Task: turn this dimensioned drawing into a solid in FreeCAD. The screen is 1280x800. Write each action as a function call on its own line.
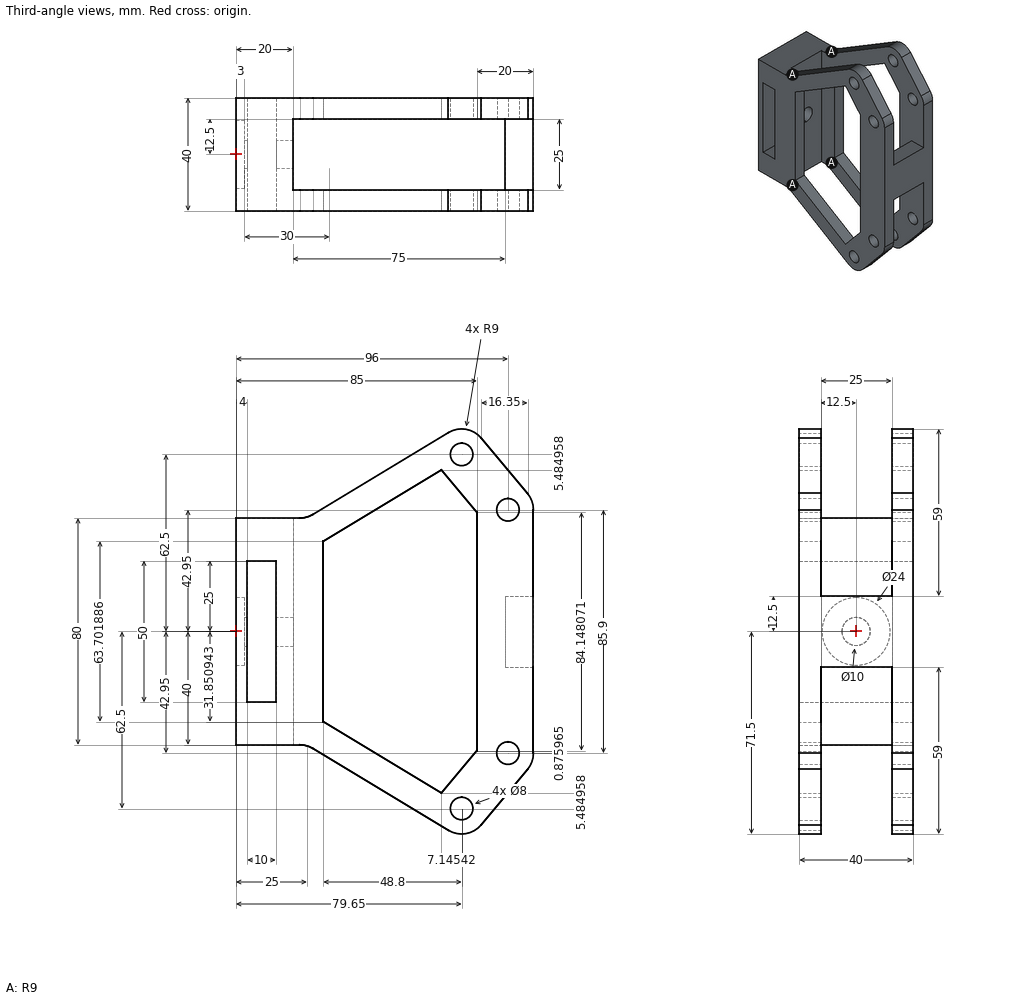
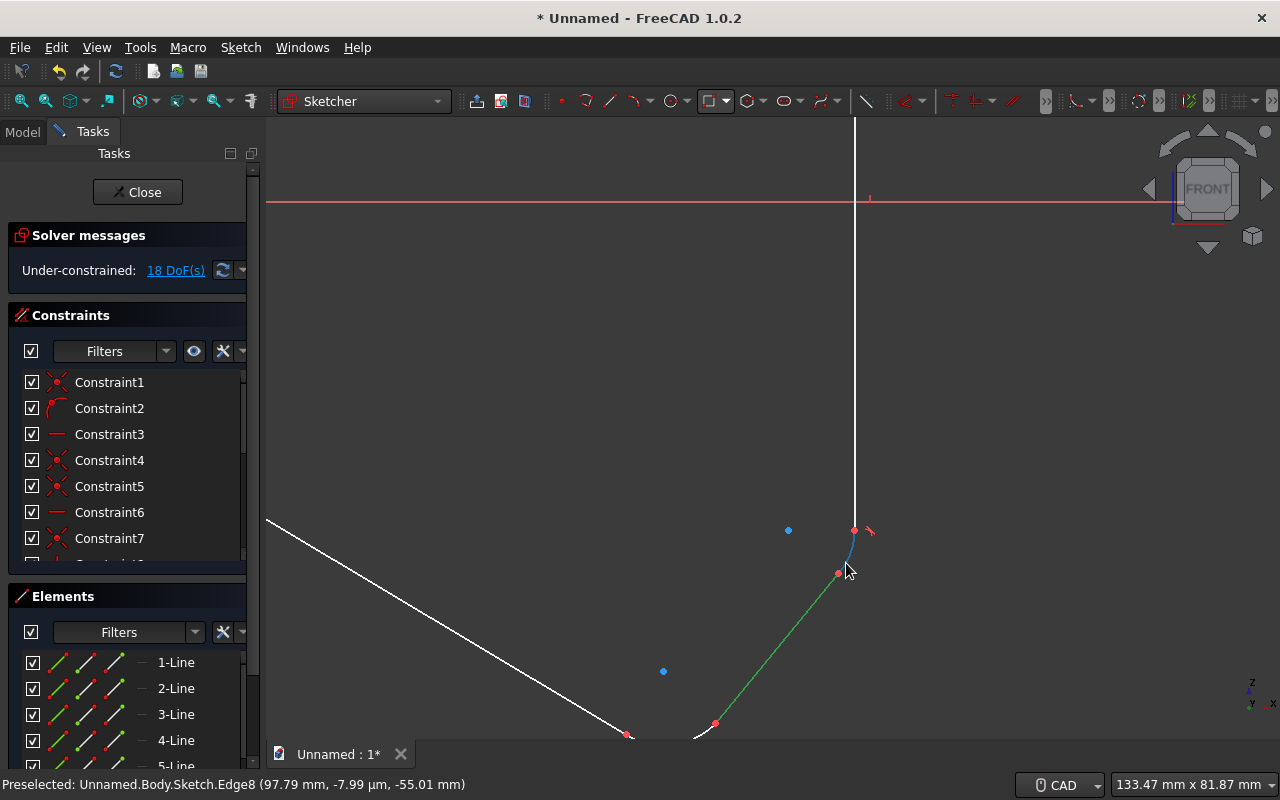
click(846, 562)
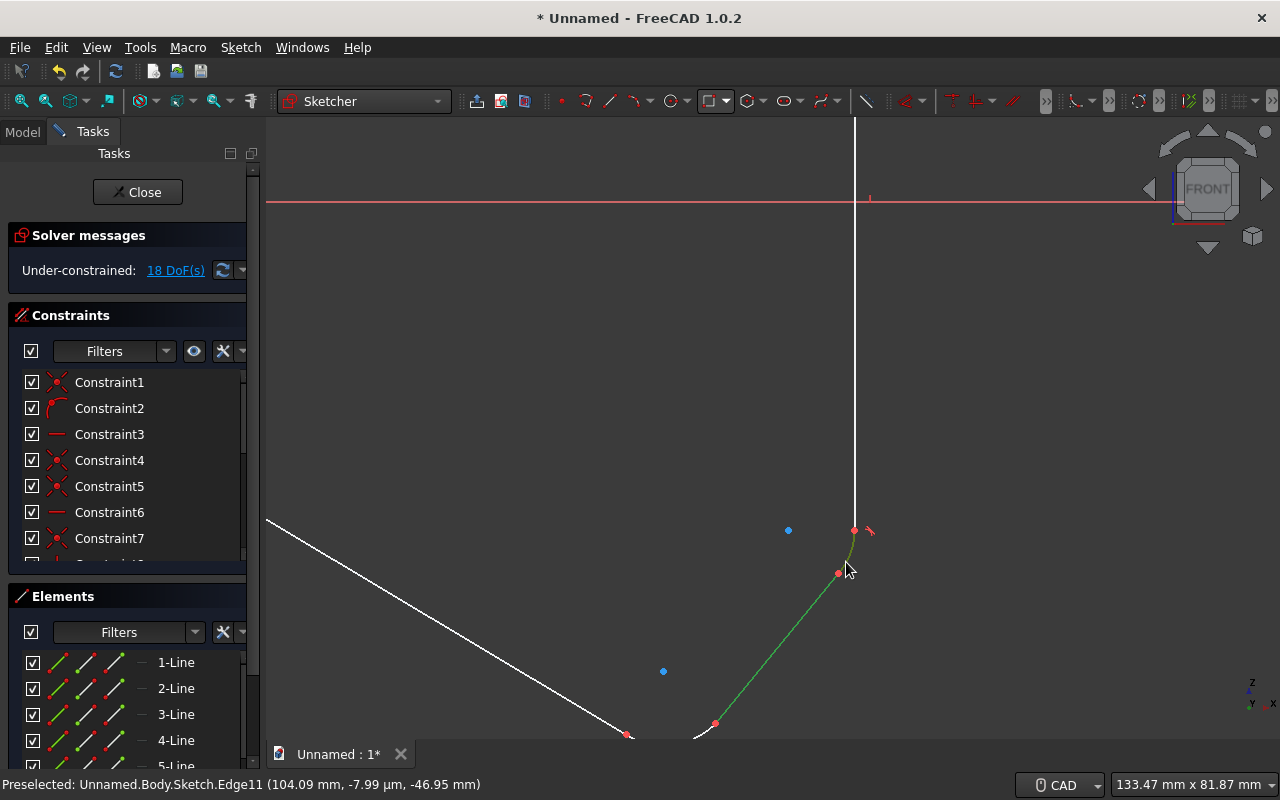
key(t)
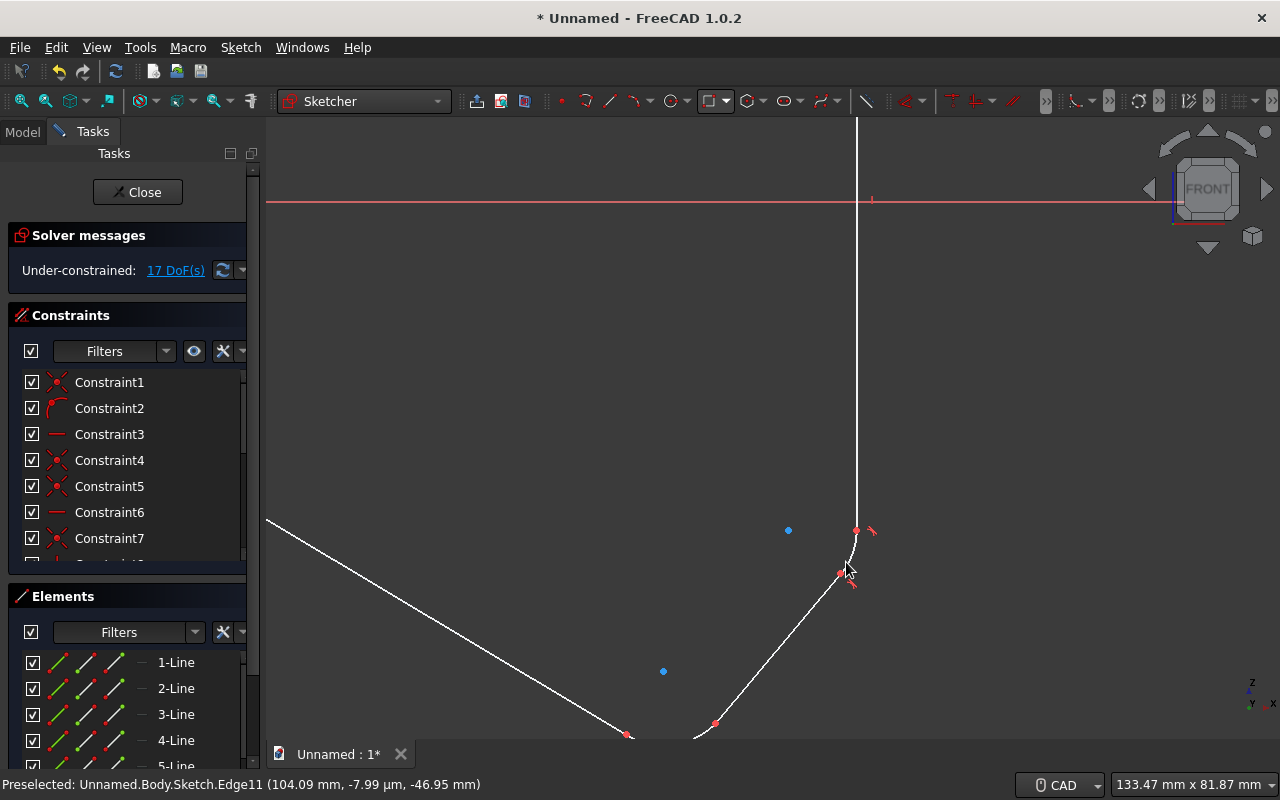
click(803, 619)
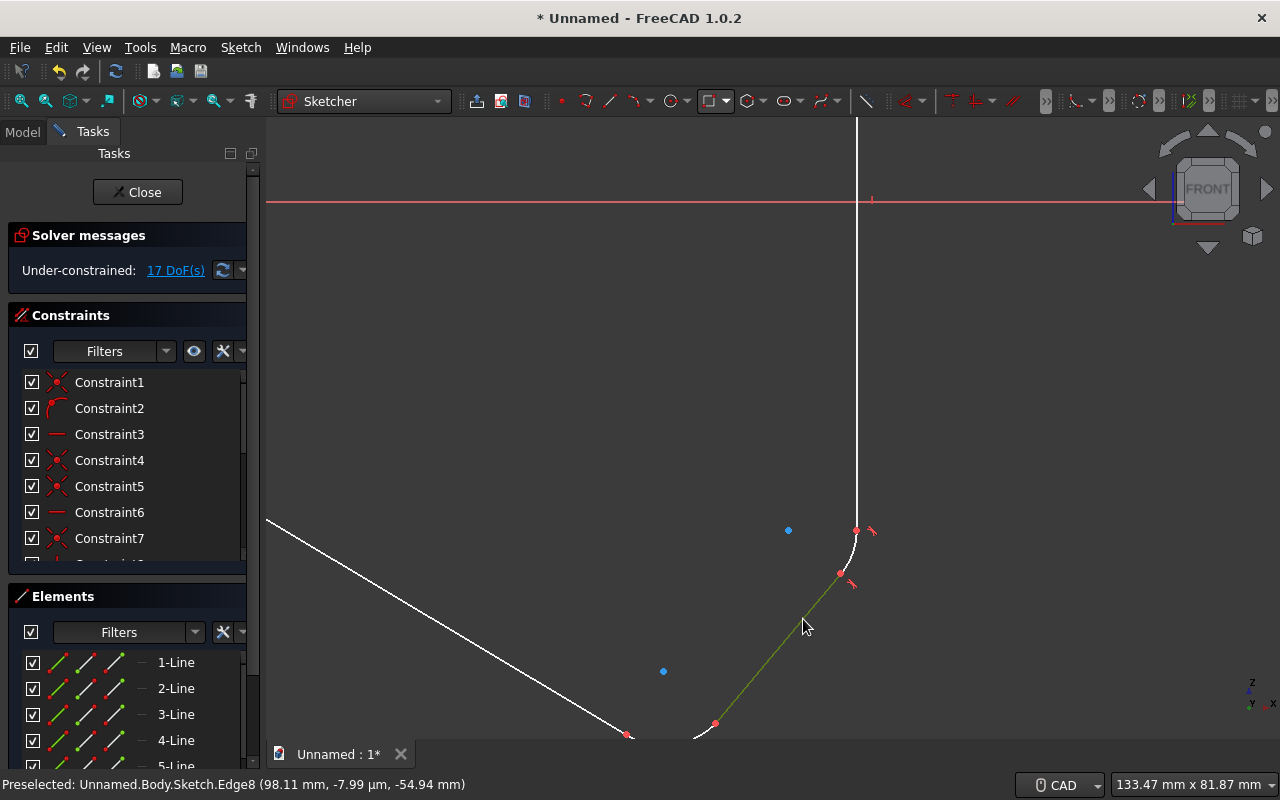
scroll(849, 559, down, 5)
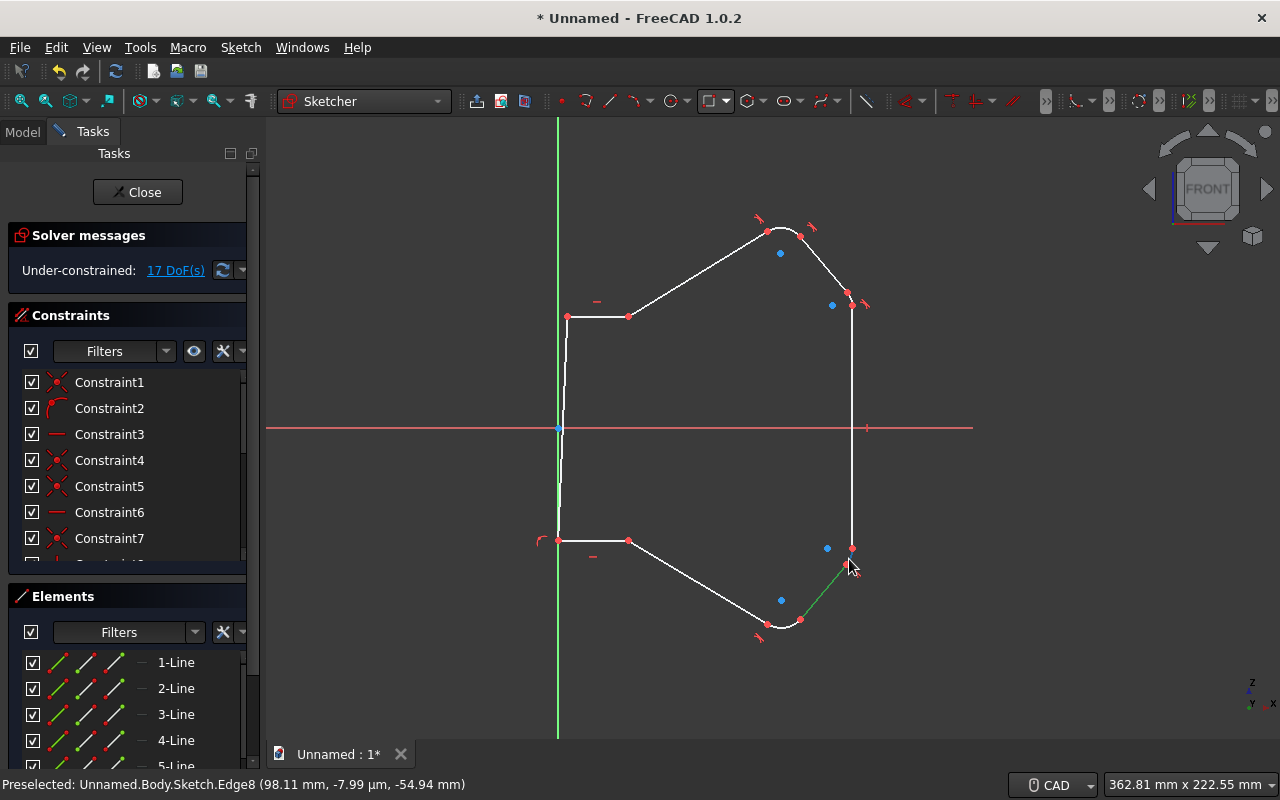
scroll(777, 628, up, 2)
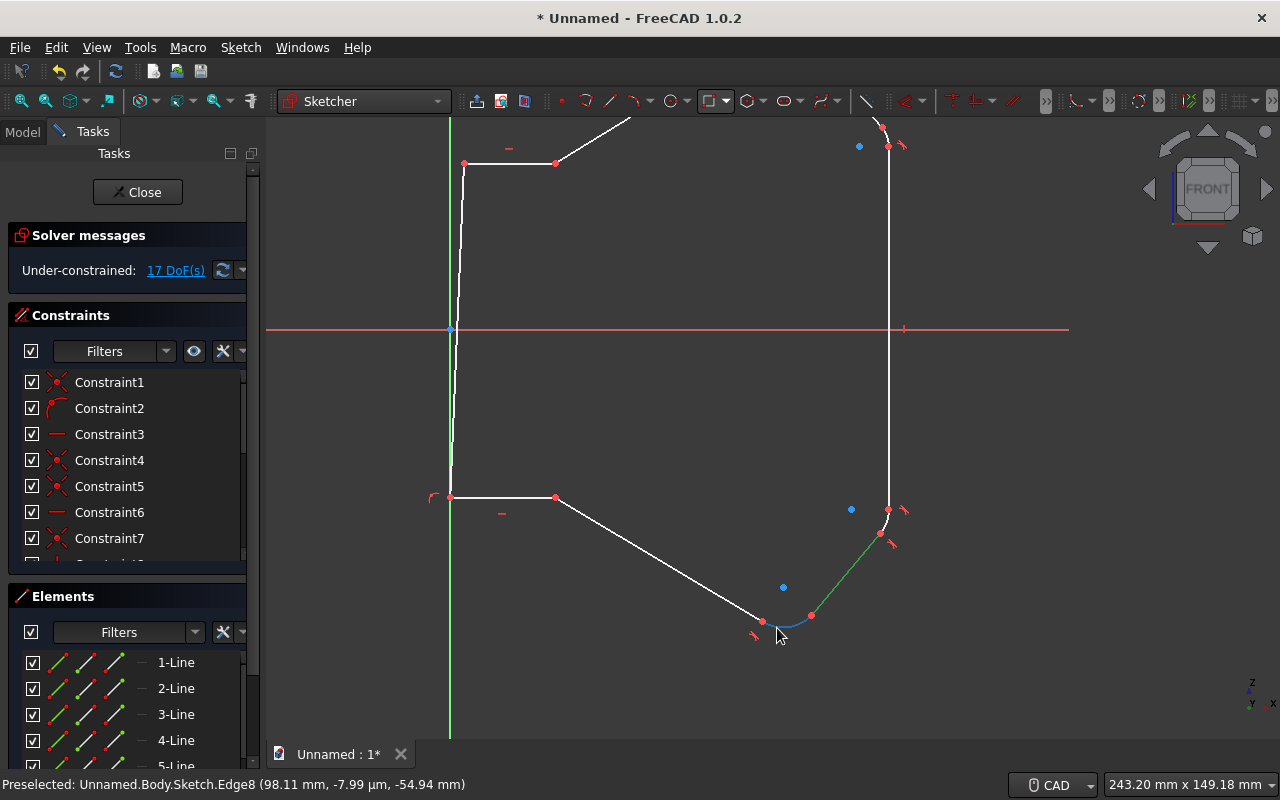
click(777, 627)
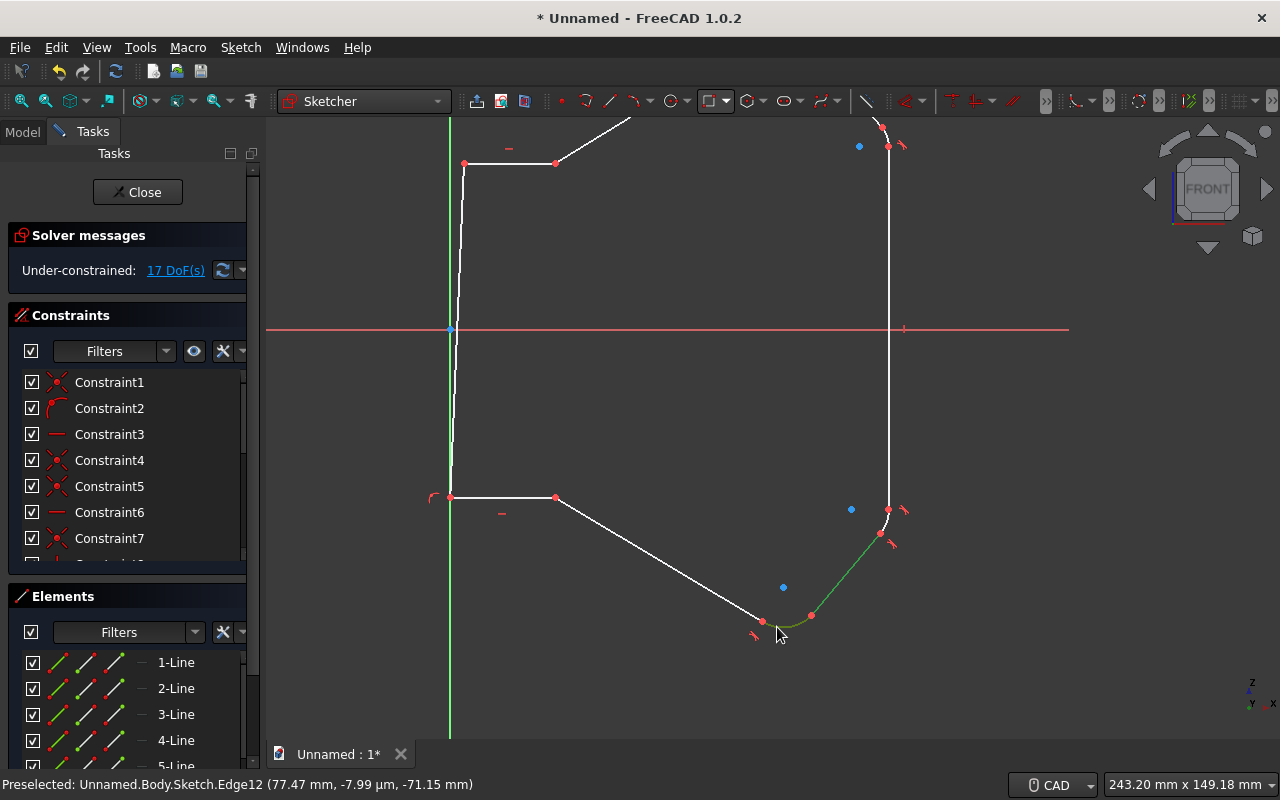
key(t)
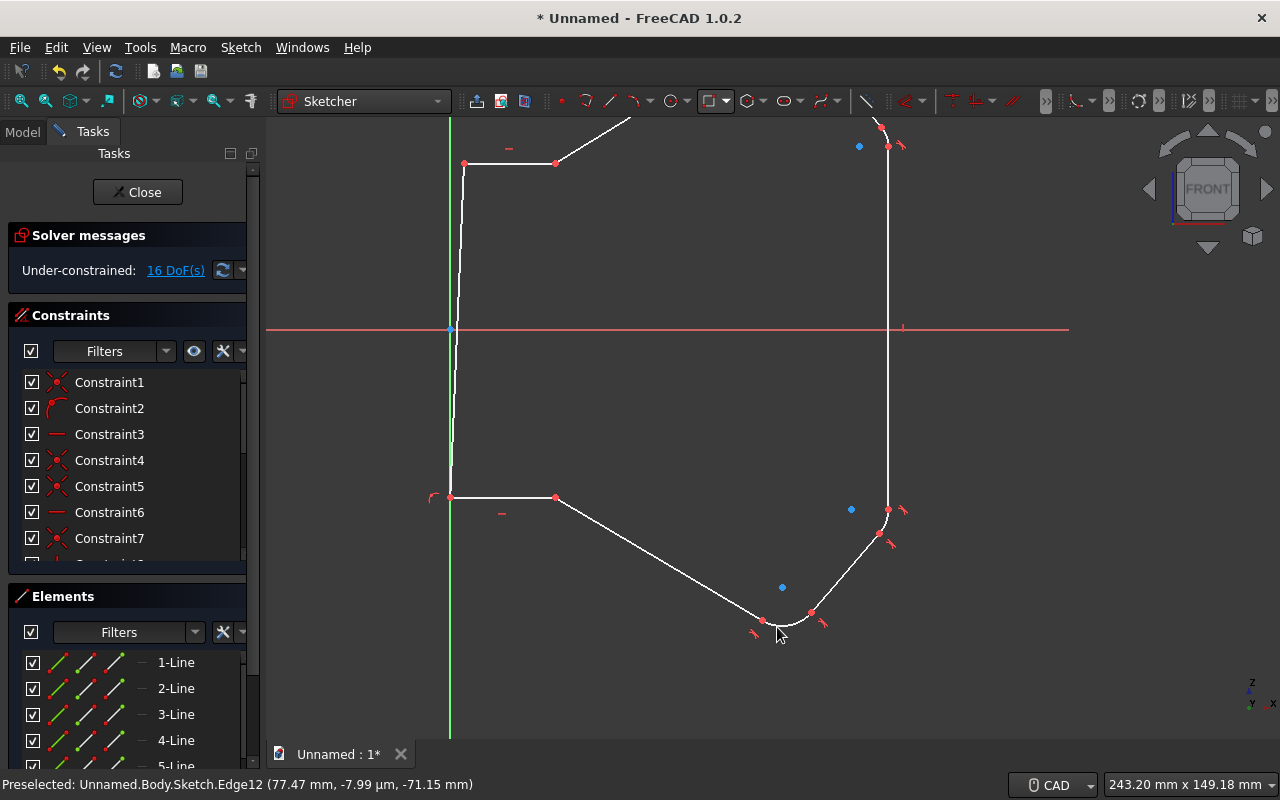
scroll(460, 264, up, 2)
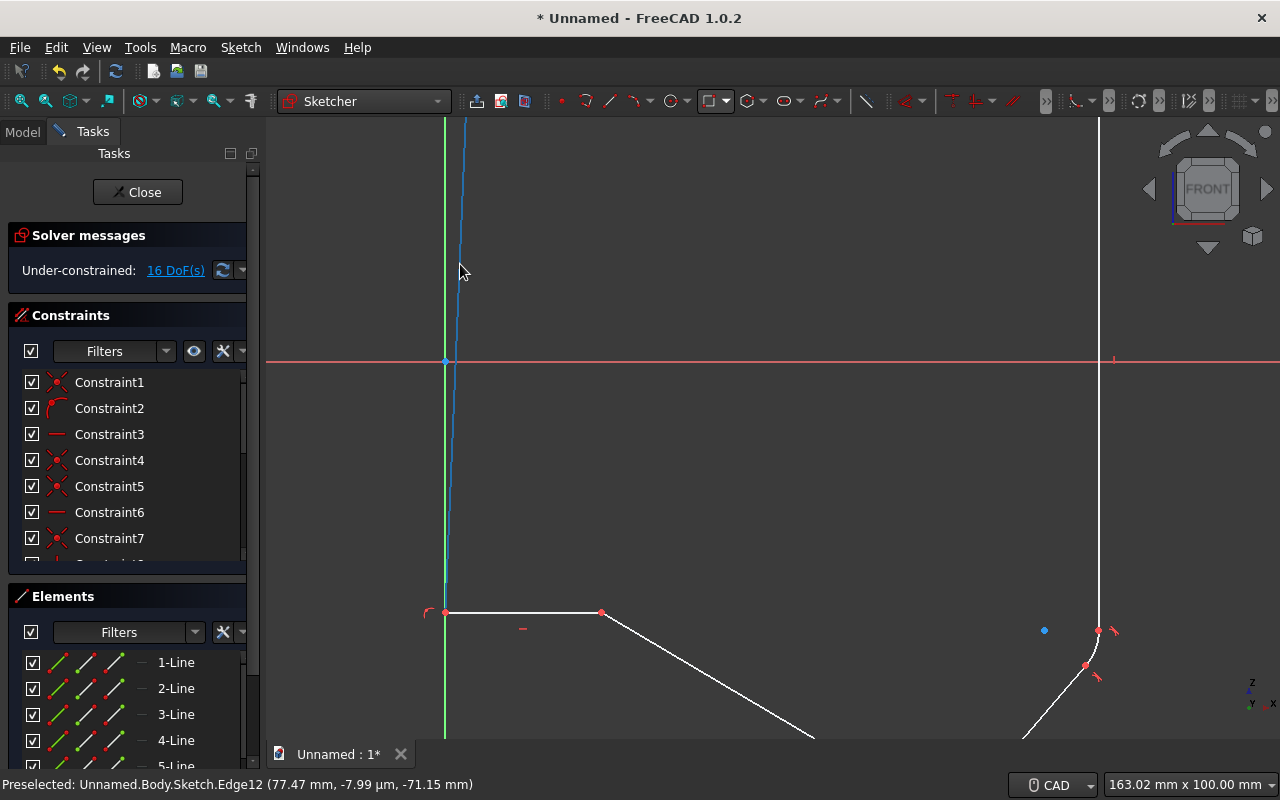
click(460, 264)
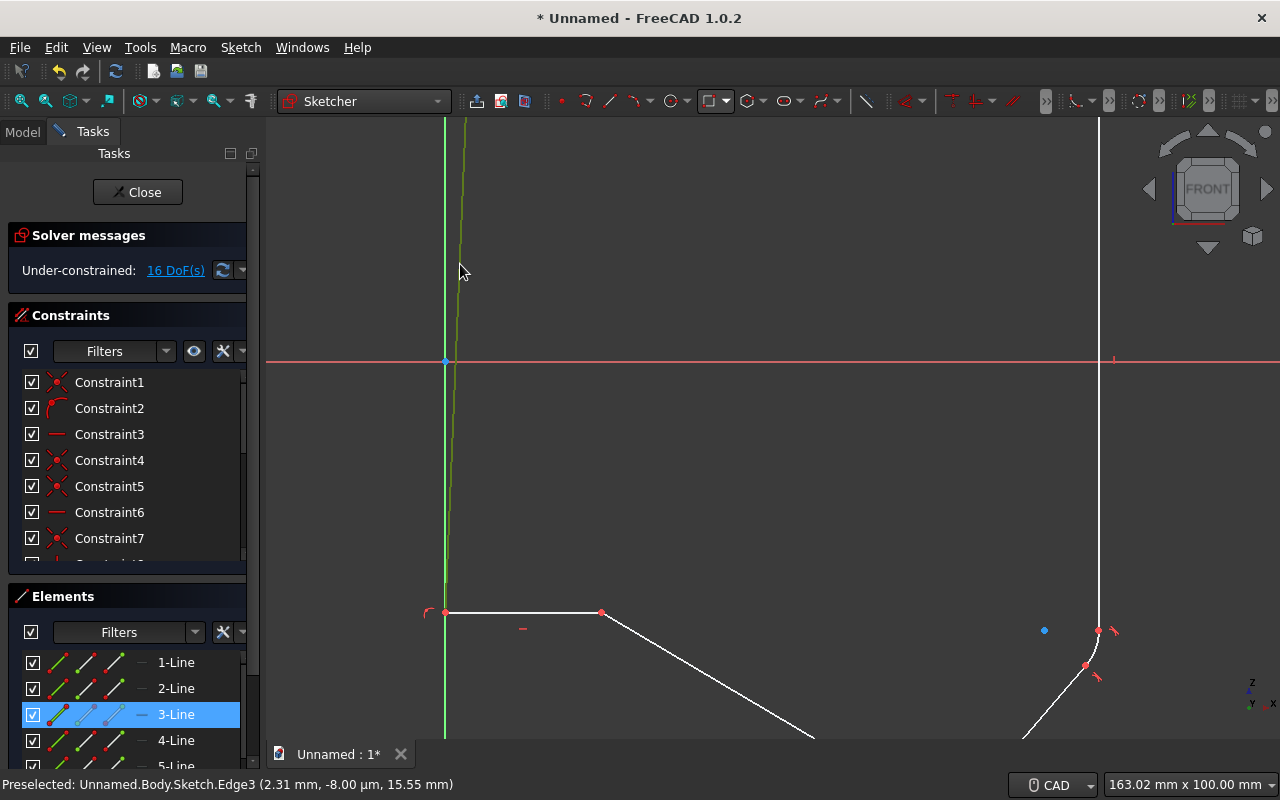
key(v)